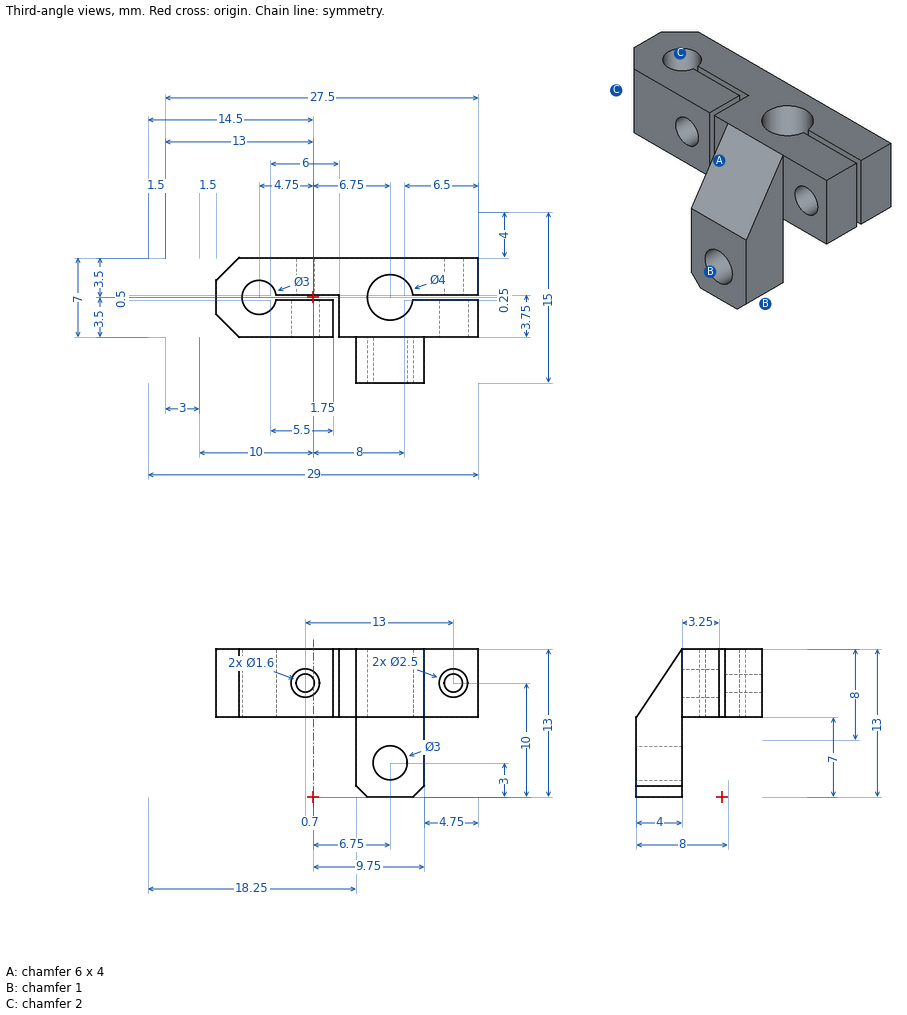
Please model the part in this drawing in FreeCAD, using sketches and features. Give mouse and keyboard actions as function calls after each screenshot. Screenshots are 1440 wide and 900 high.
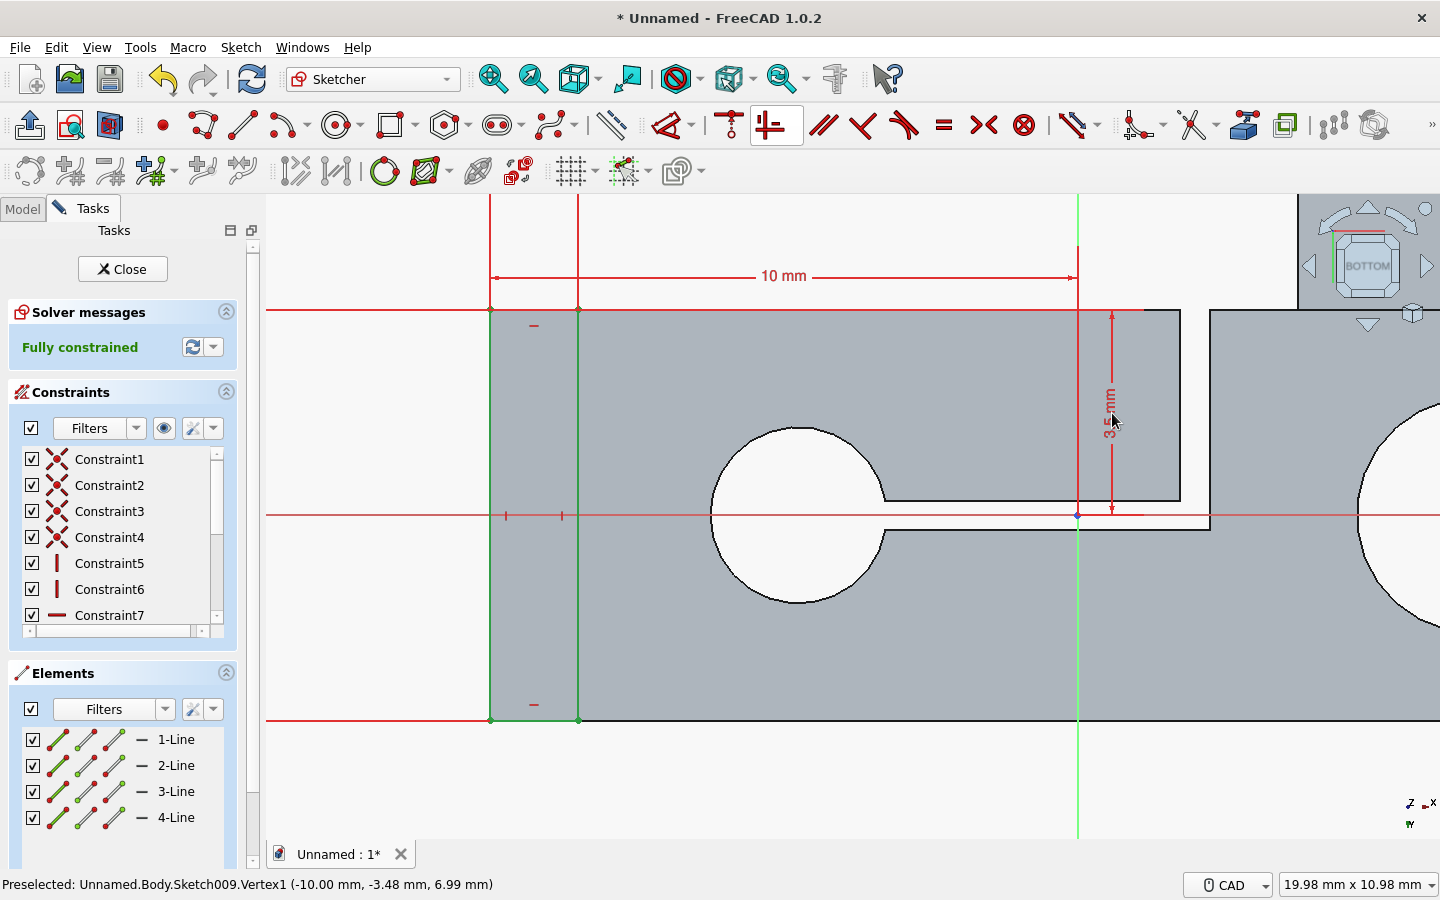
click(123, 269)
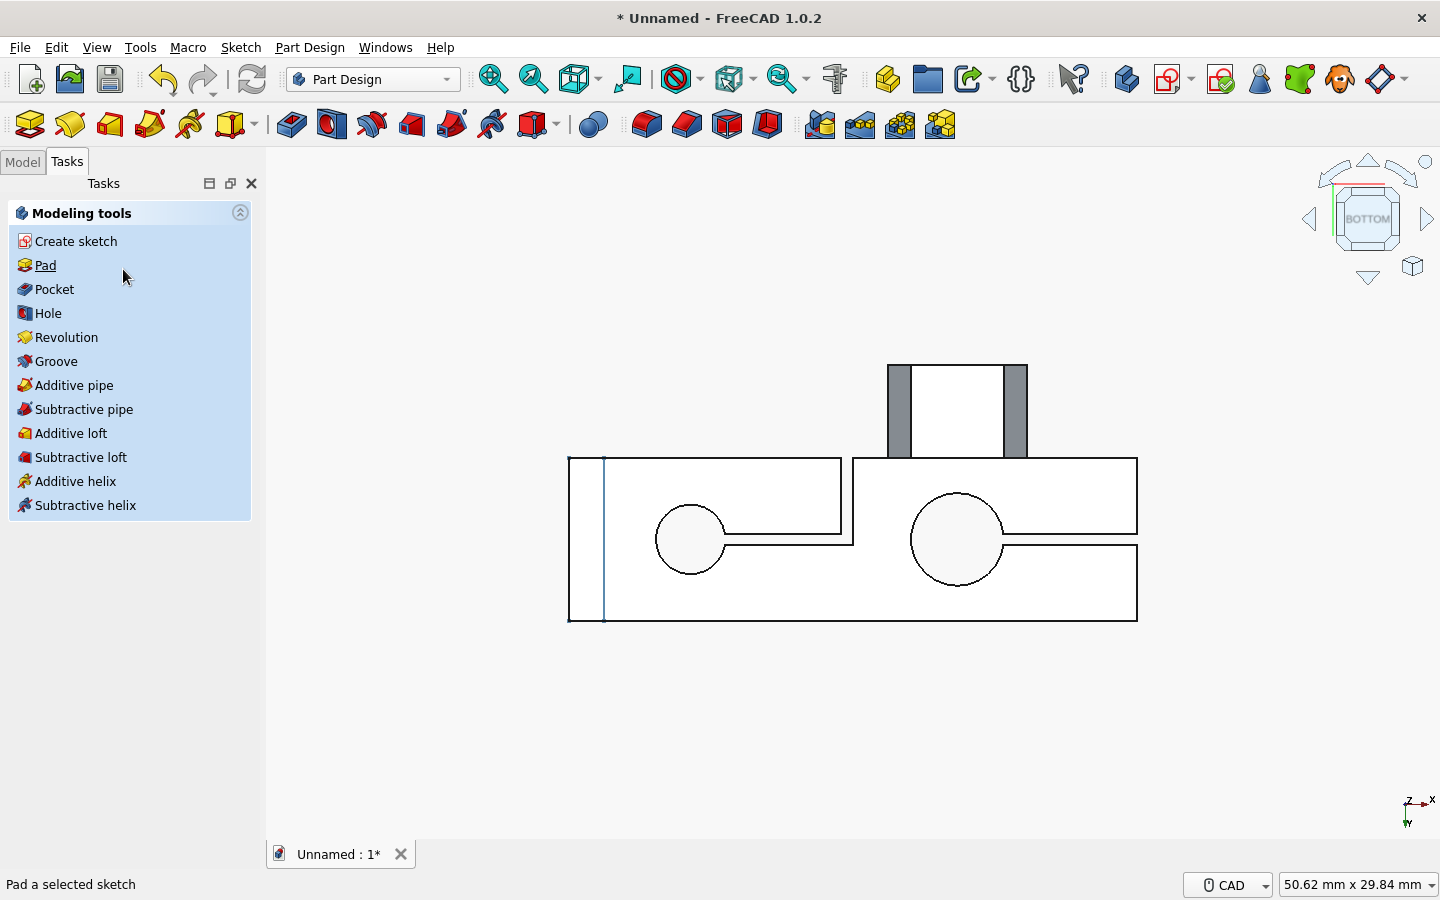
click(292, 124)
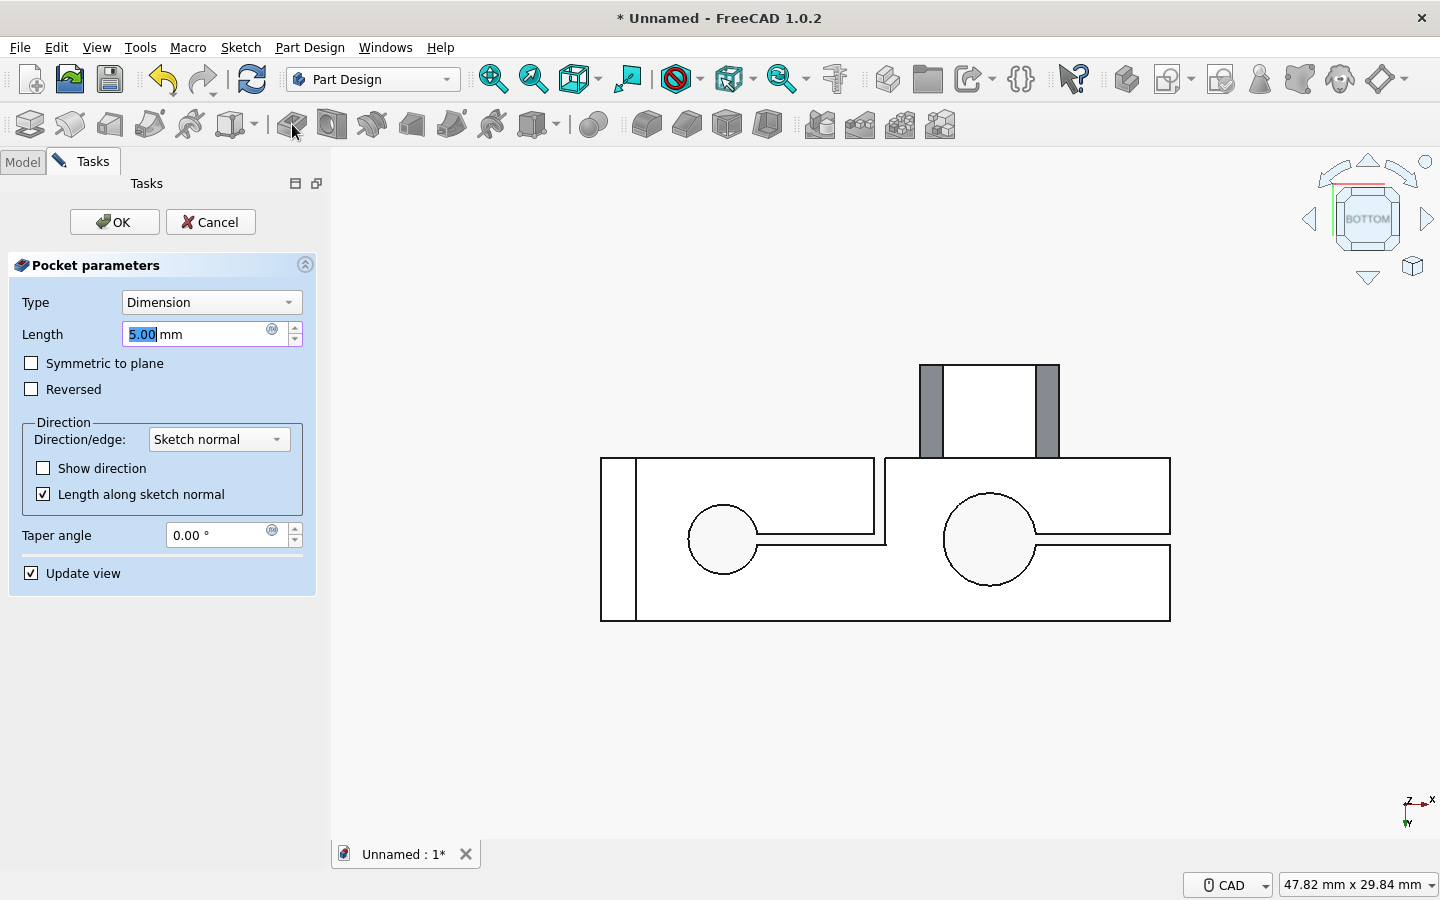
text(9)
key(Tab)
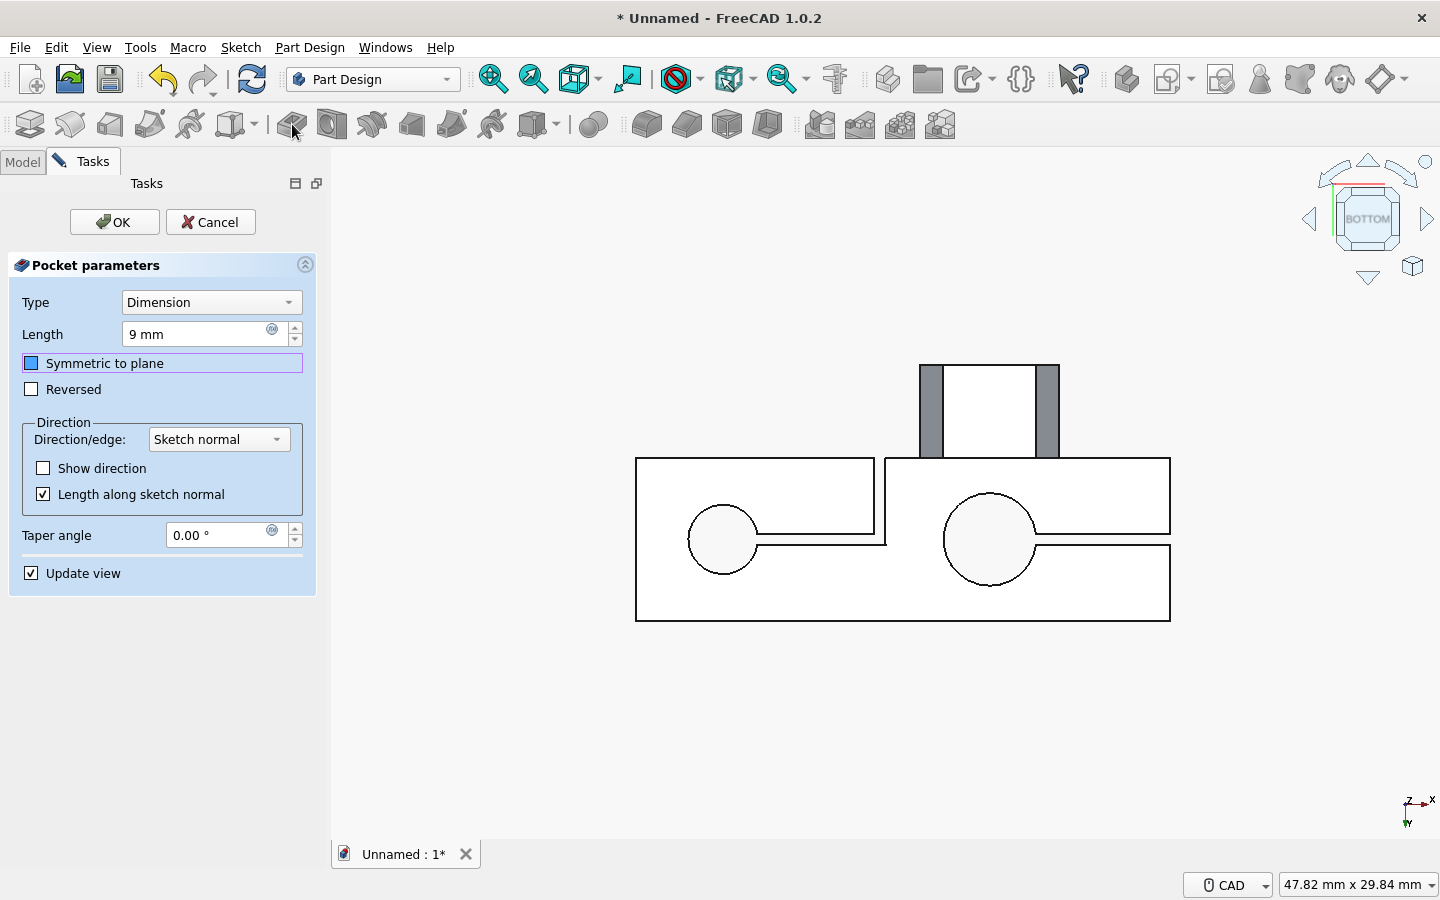
click(115, 222)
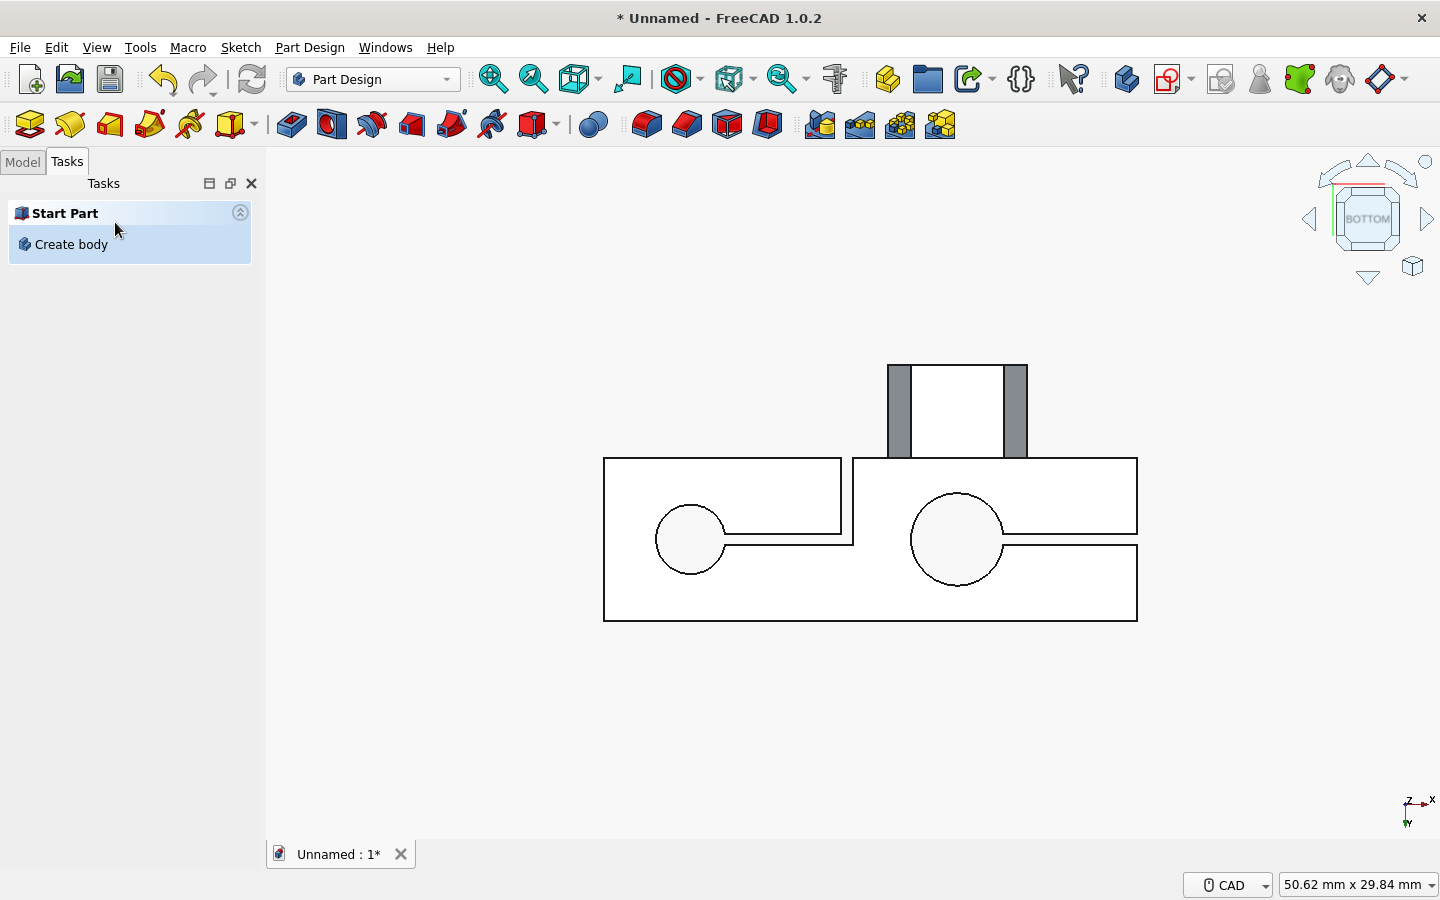
key(0)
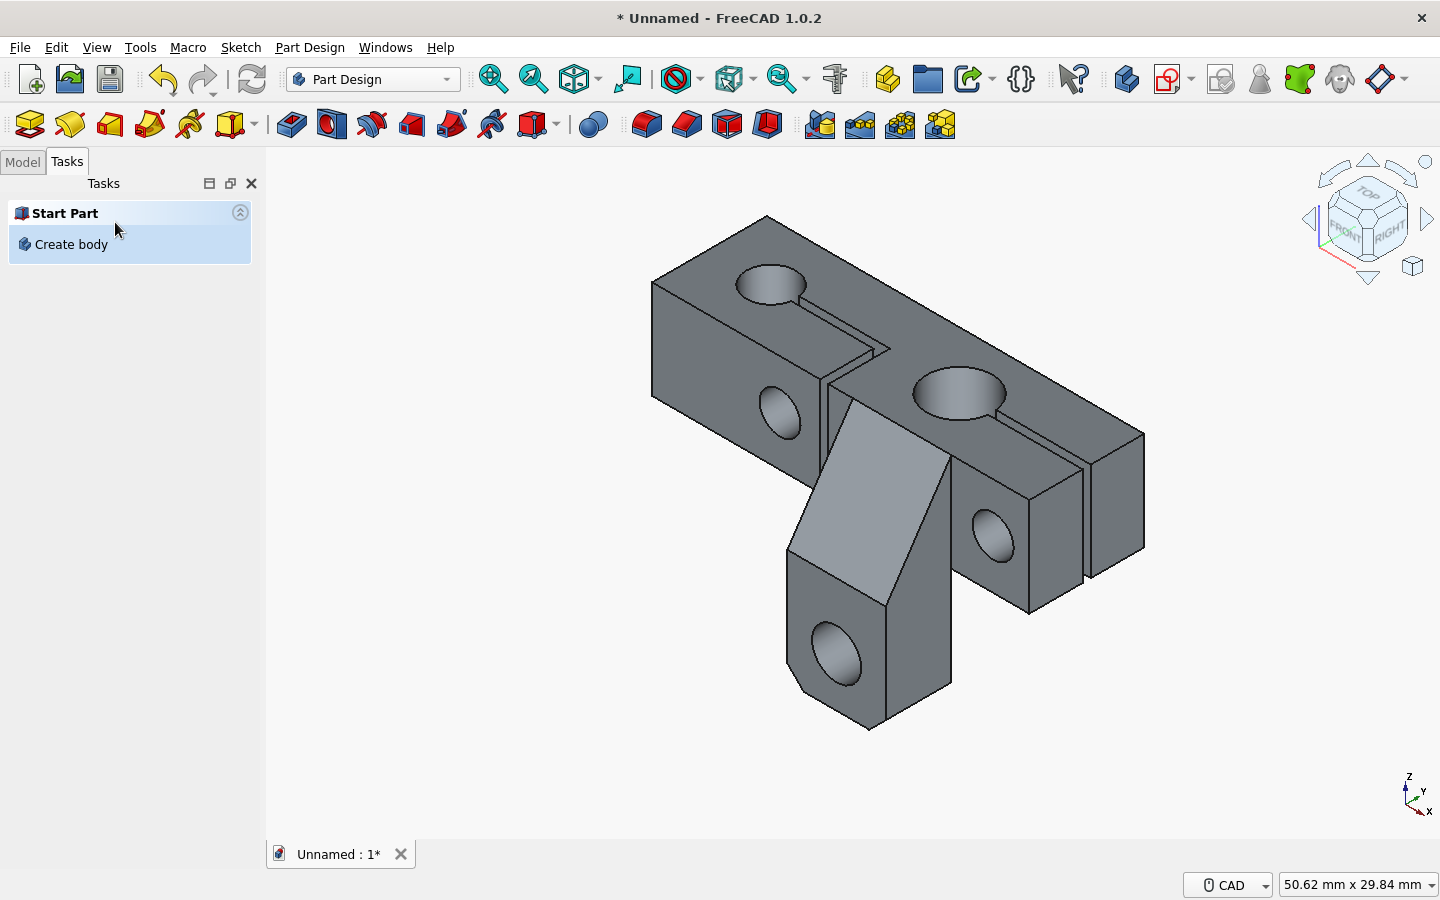
key(2)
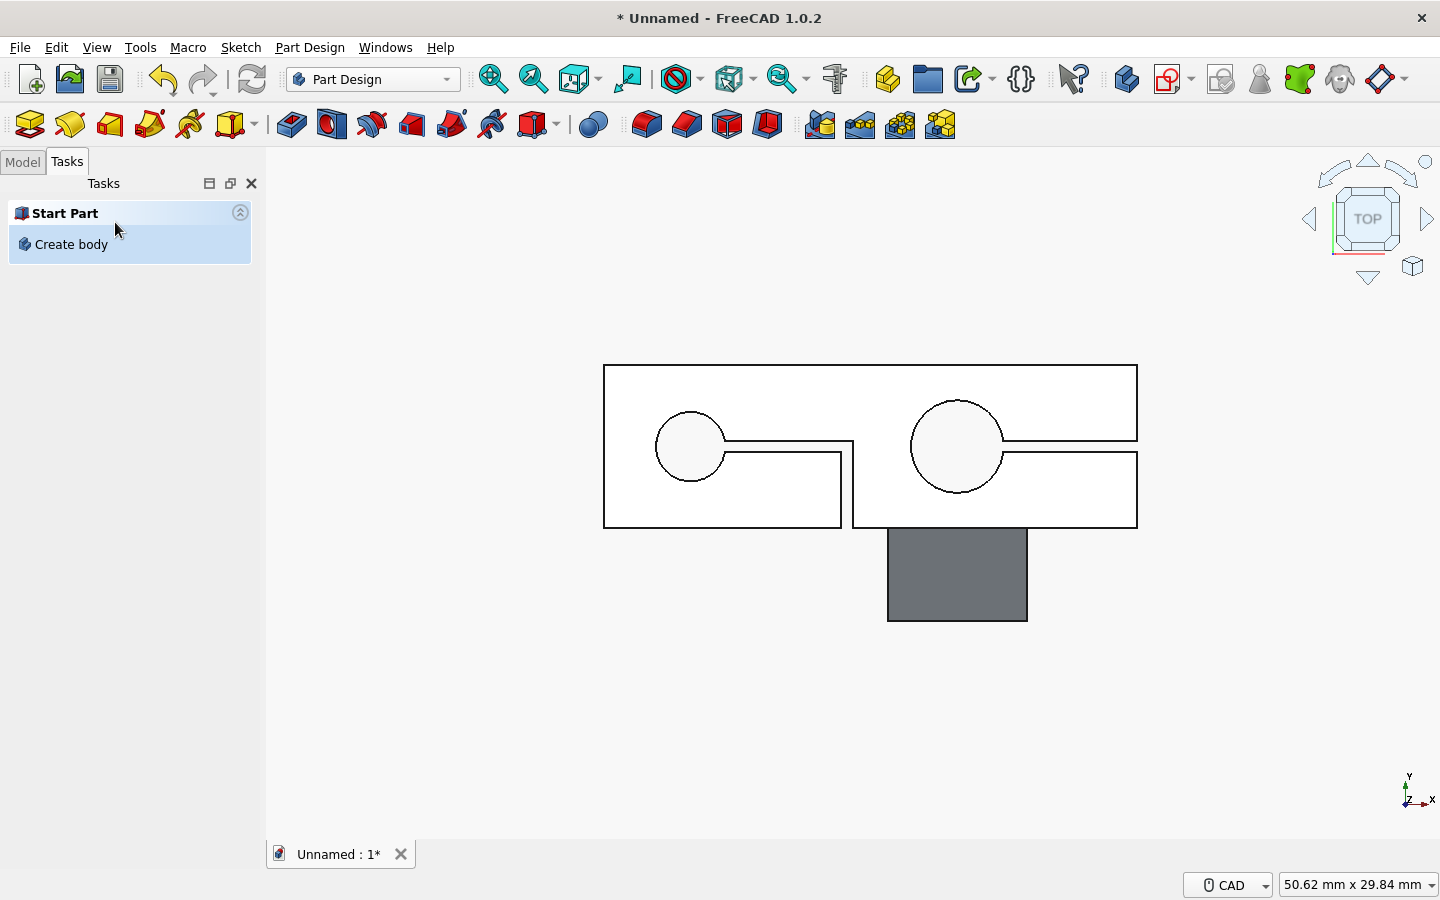
key(1)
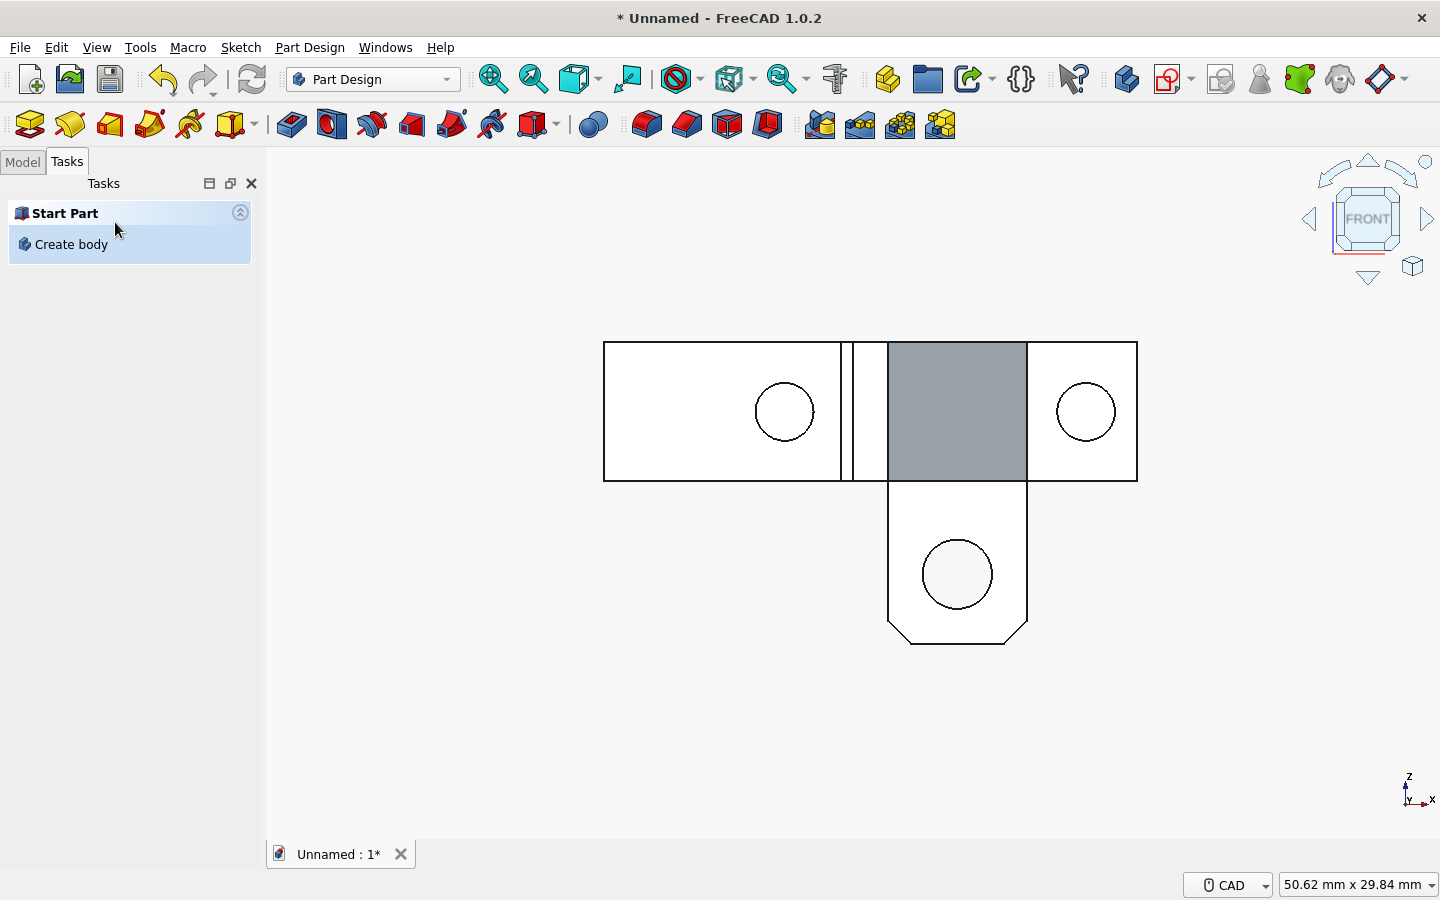
click(604, 411)